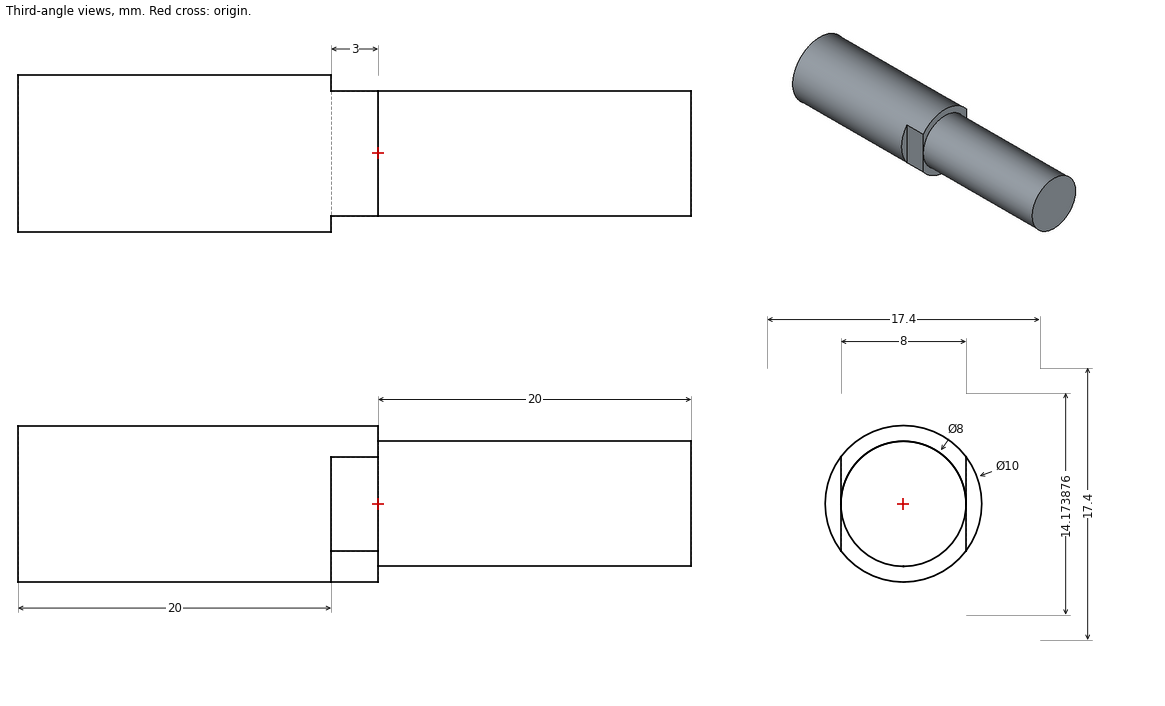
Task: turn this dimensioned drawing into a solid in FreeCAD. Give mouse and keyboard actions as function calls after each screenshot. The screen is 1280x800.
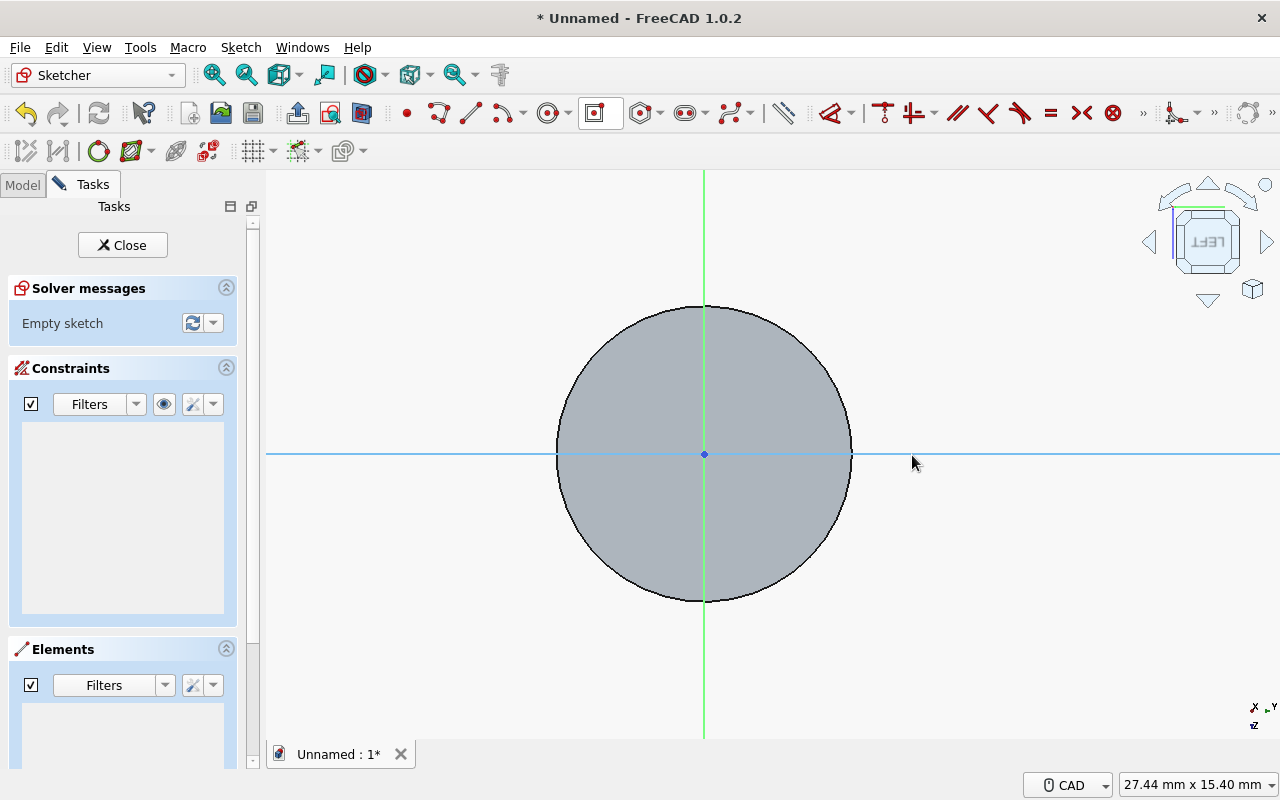
click(548, 114)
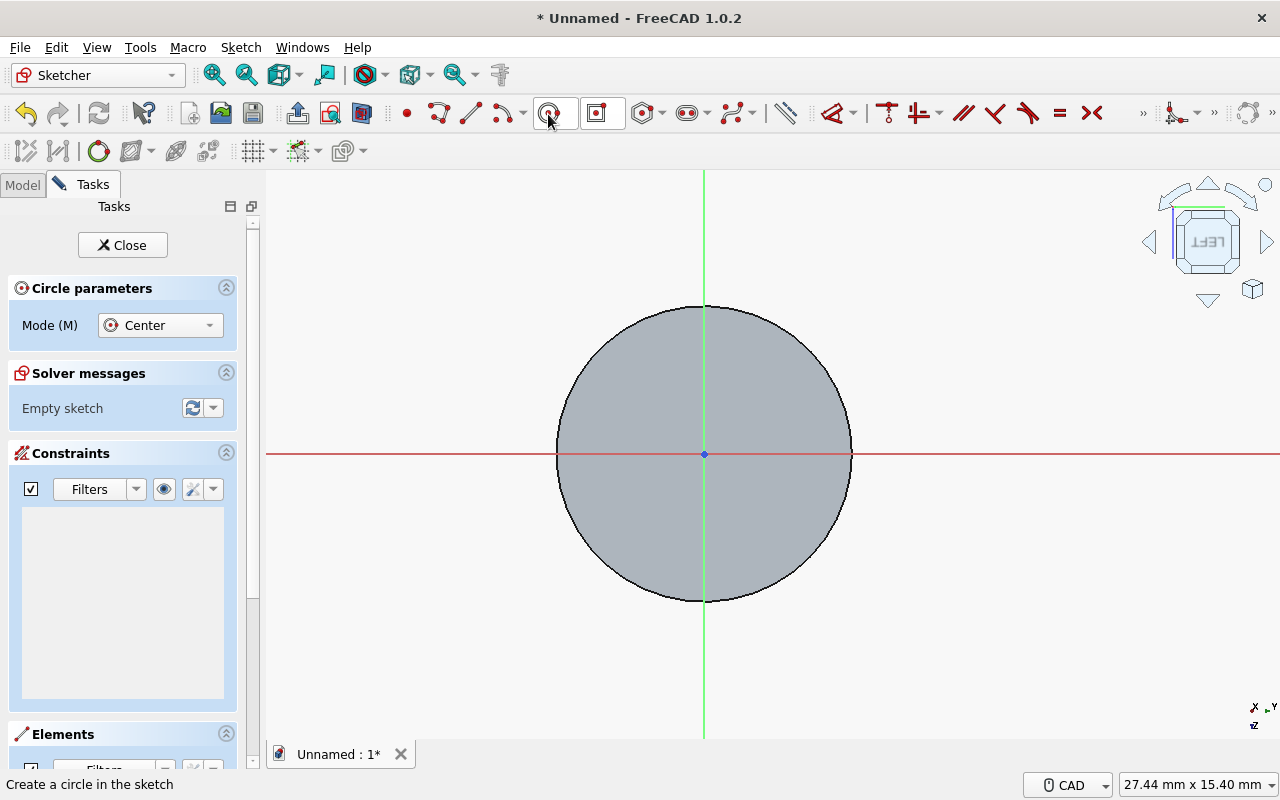
click(704, 454)
click(835, 323)
key(Escape)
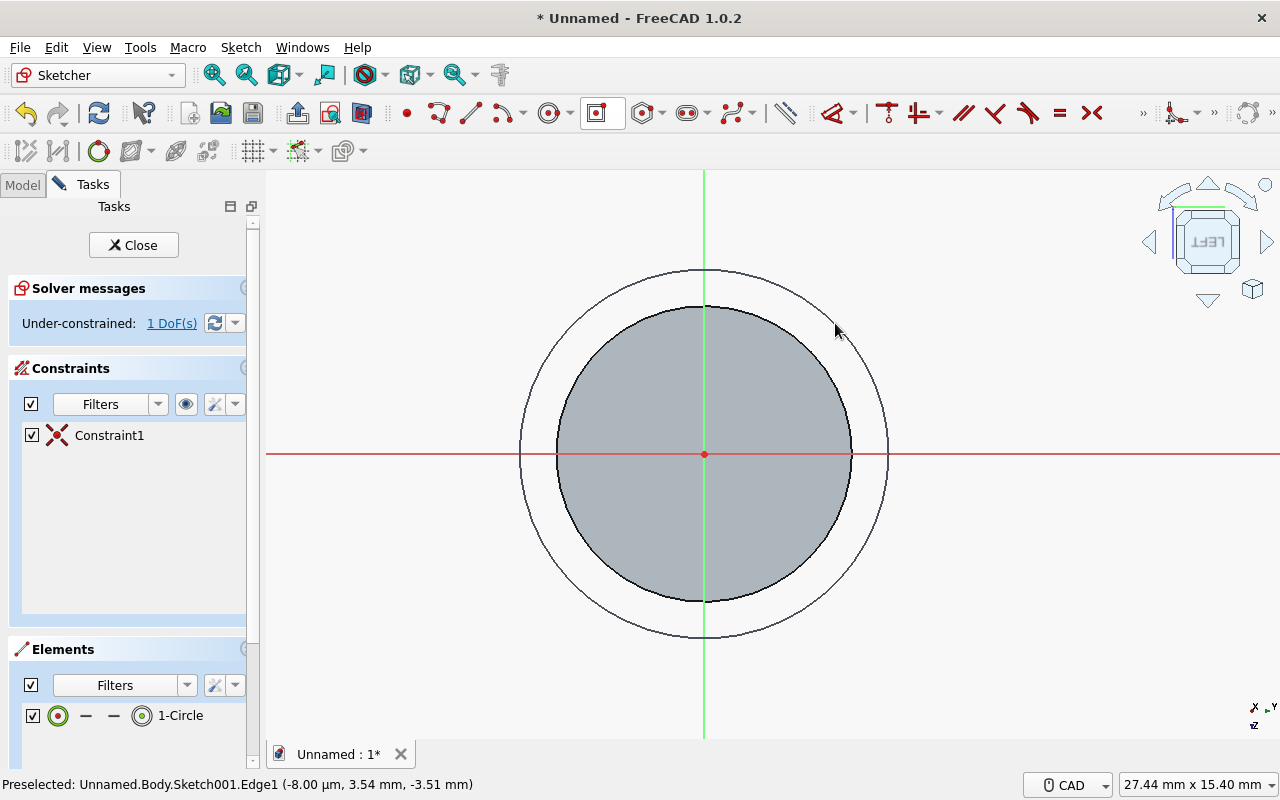
click(834, 323)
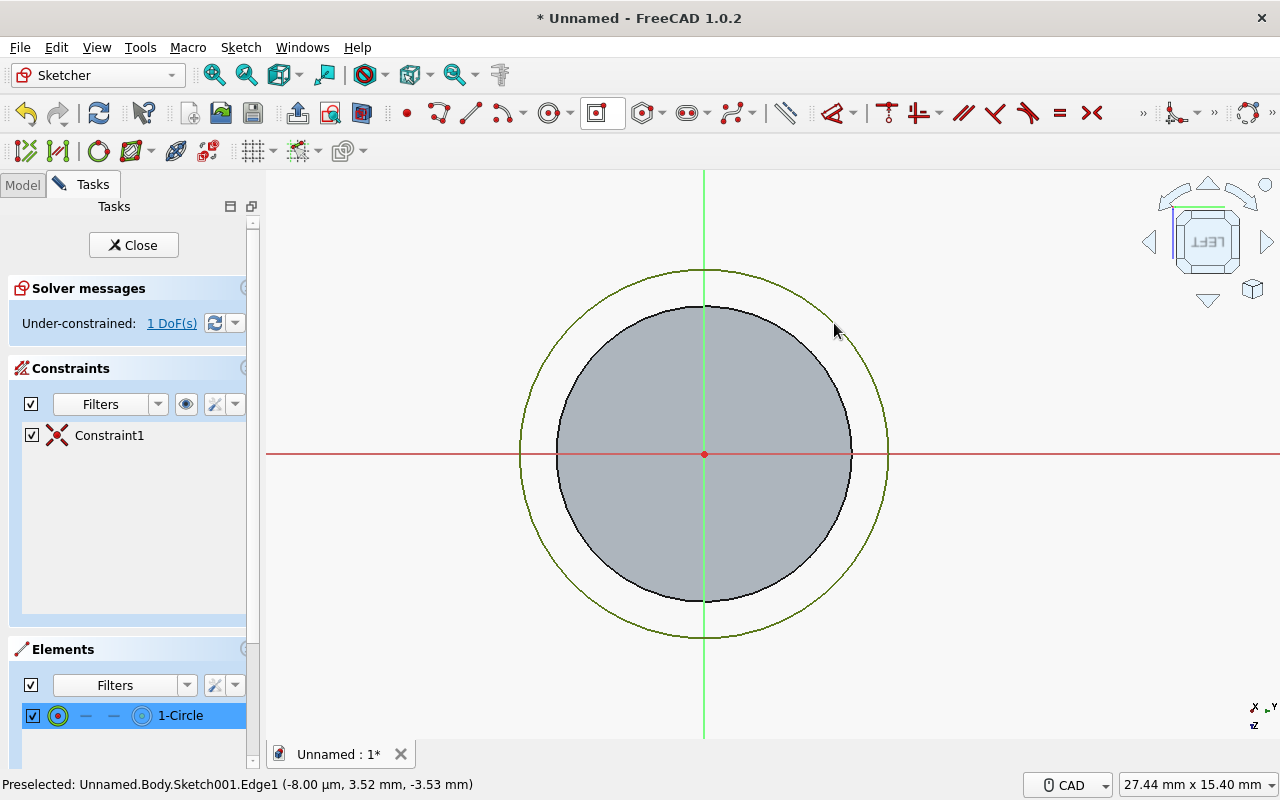
key(k)
key(o)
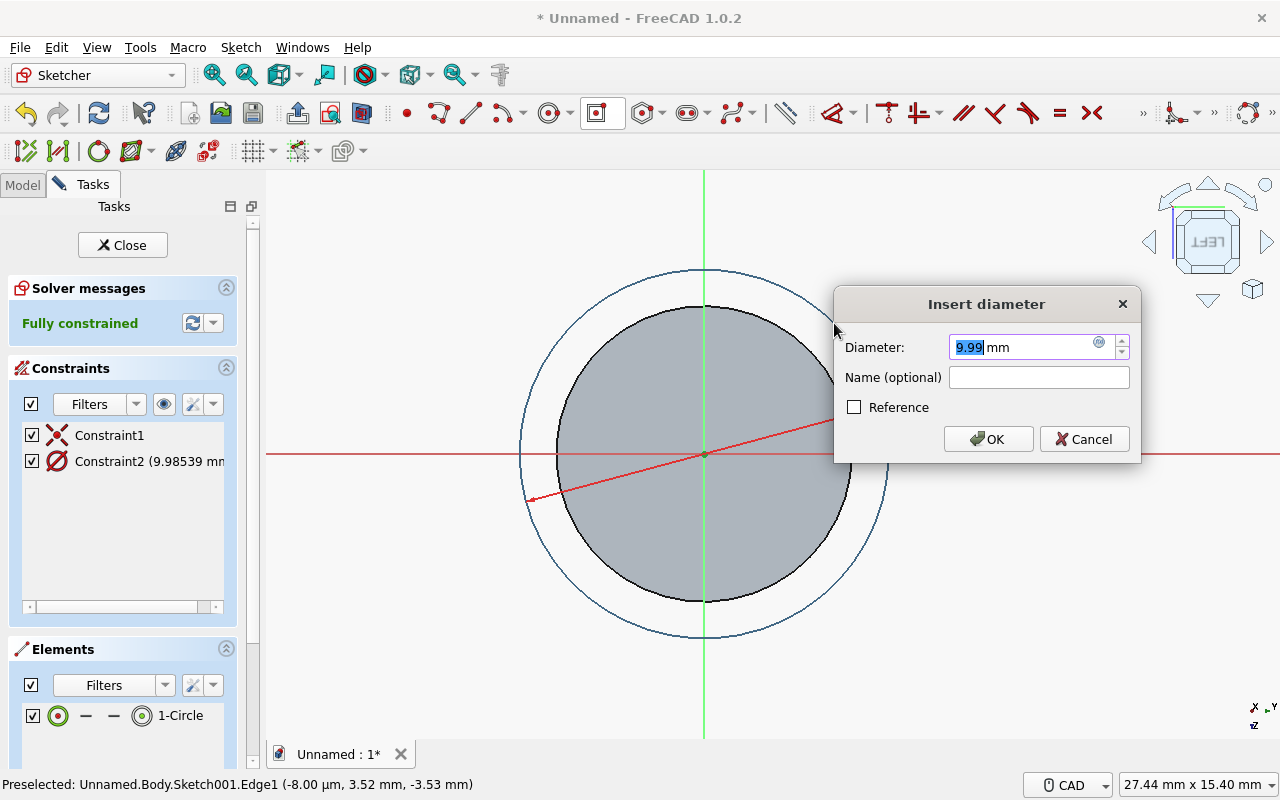
text(10)
key(Return)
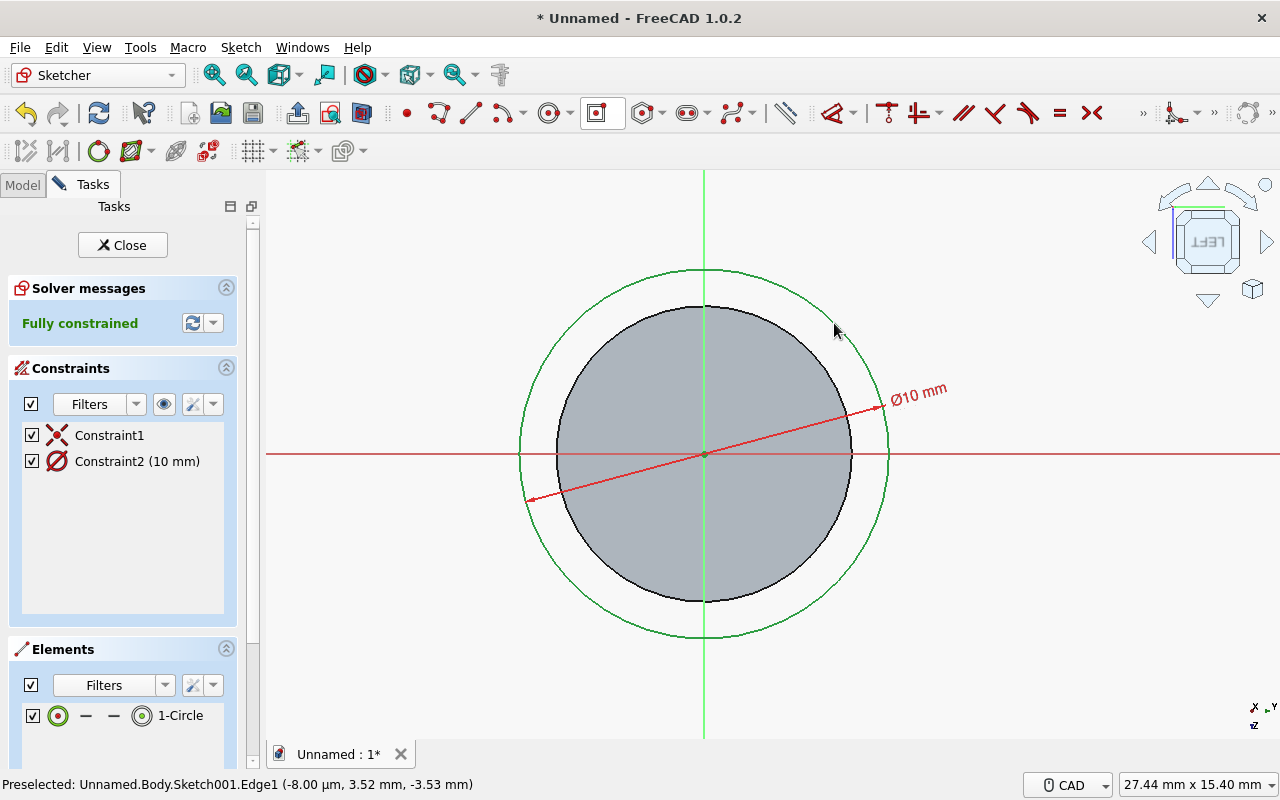
click(123, 245)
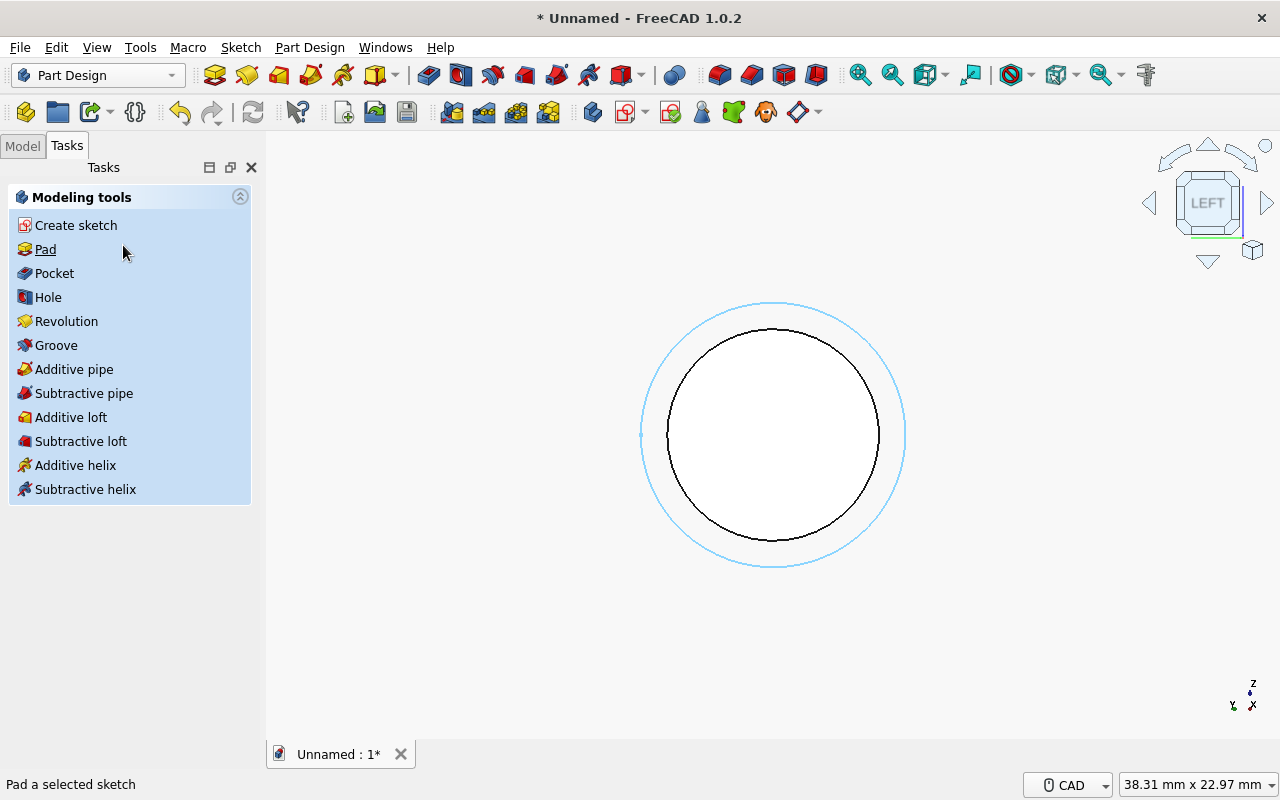
click(216, 76)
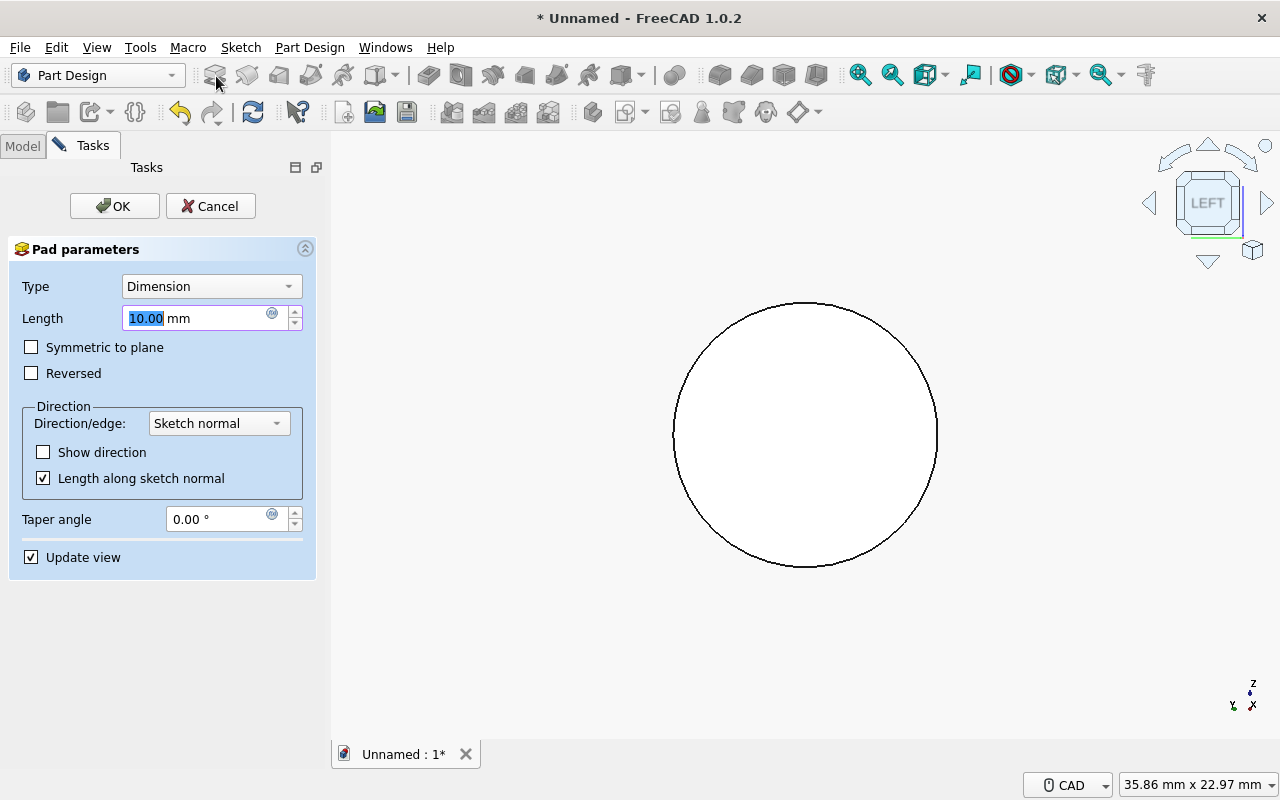
text(3)
key(Tab)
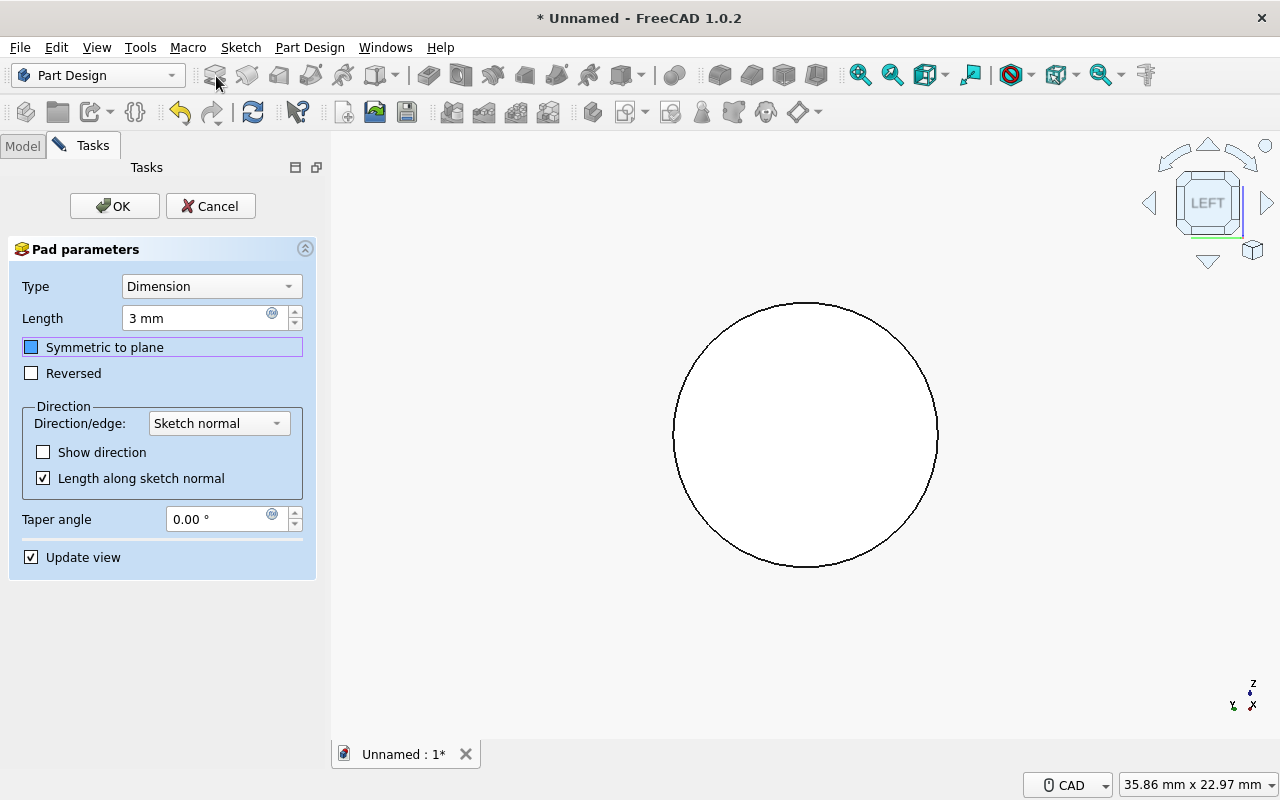
click(115, 206)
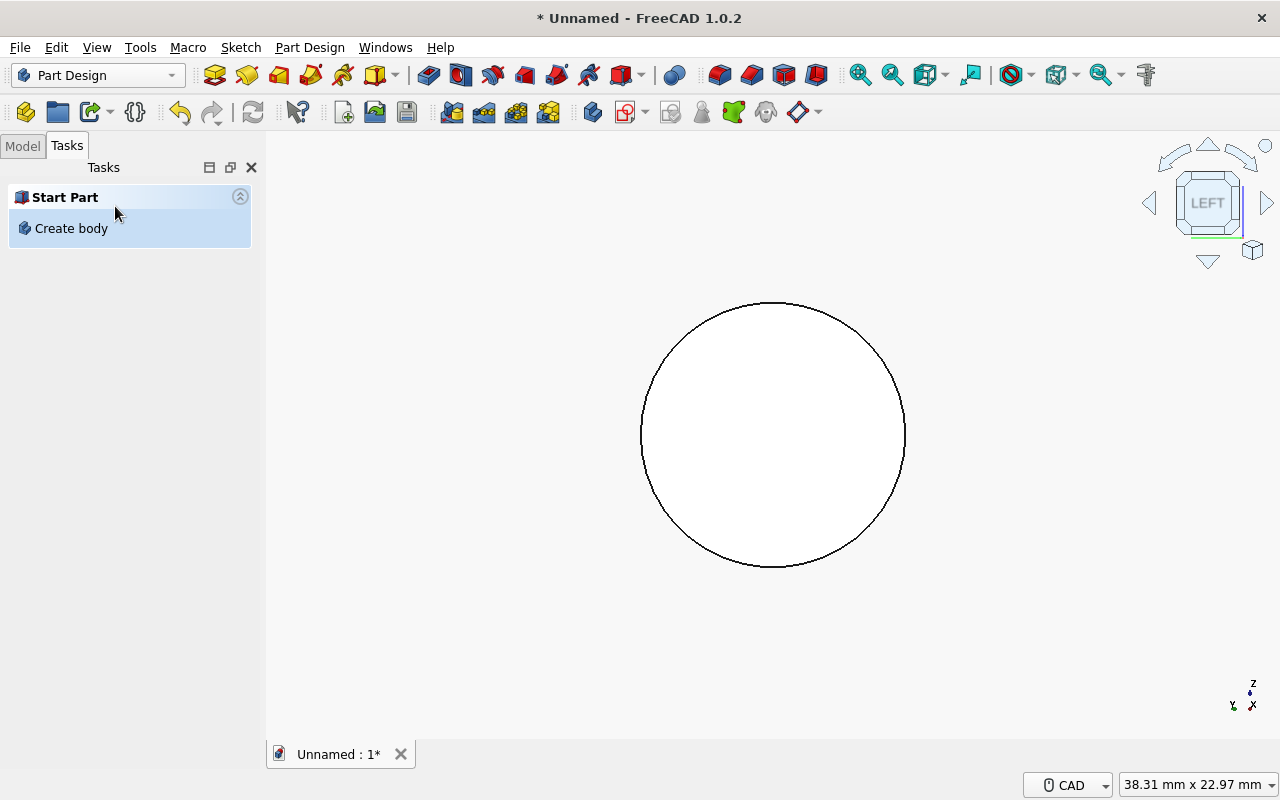
click(862, 76)